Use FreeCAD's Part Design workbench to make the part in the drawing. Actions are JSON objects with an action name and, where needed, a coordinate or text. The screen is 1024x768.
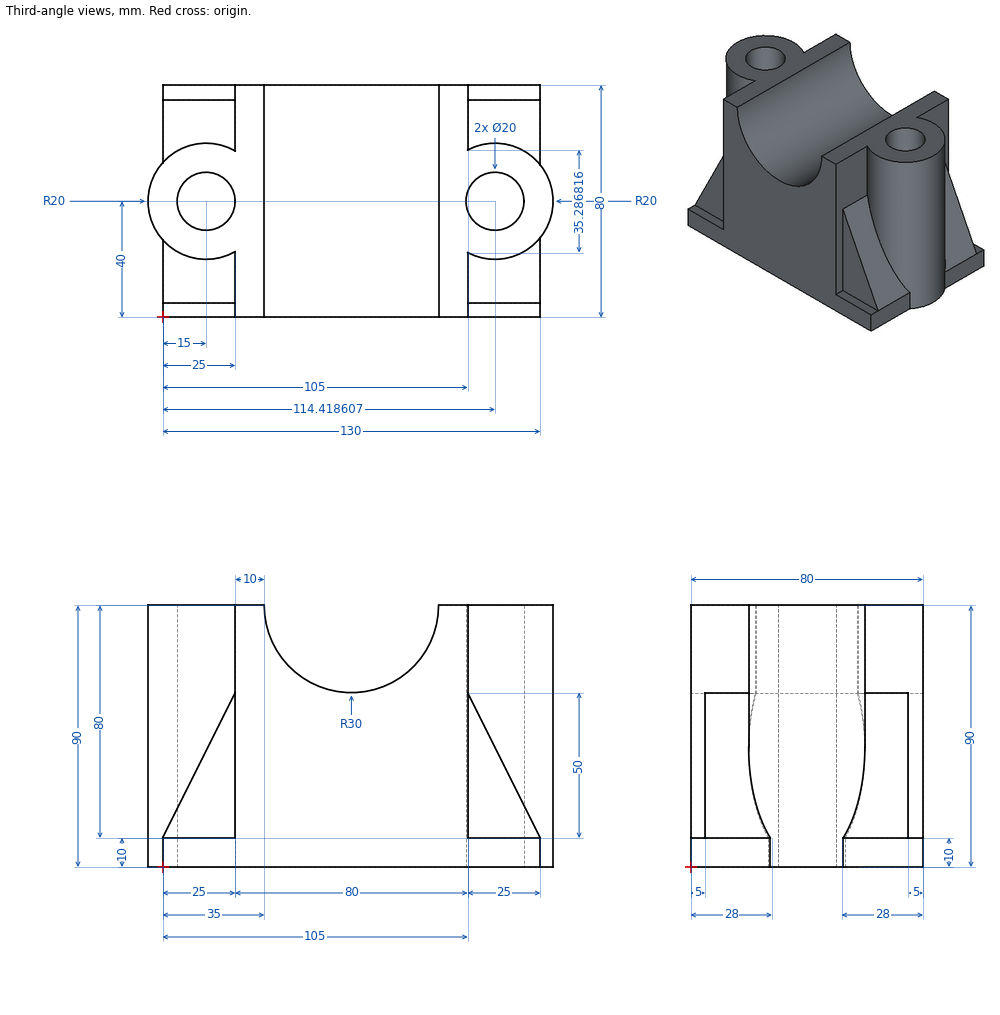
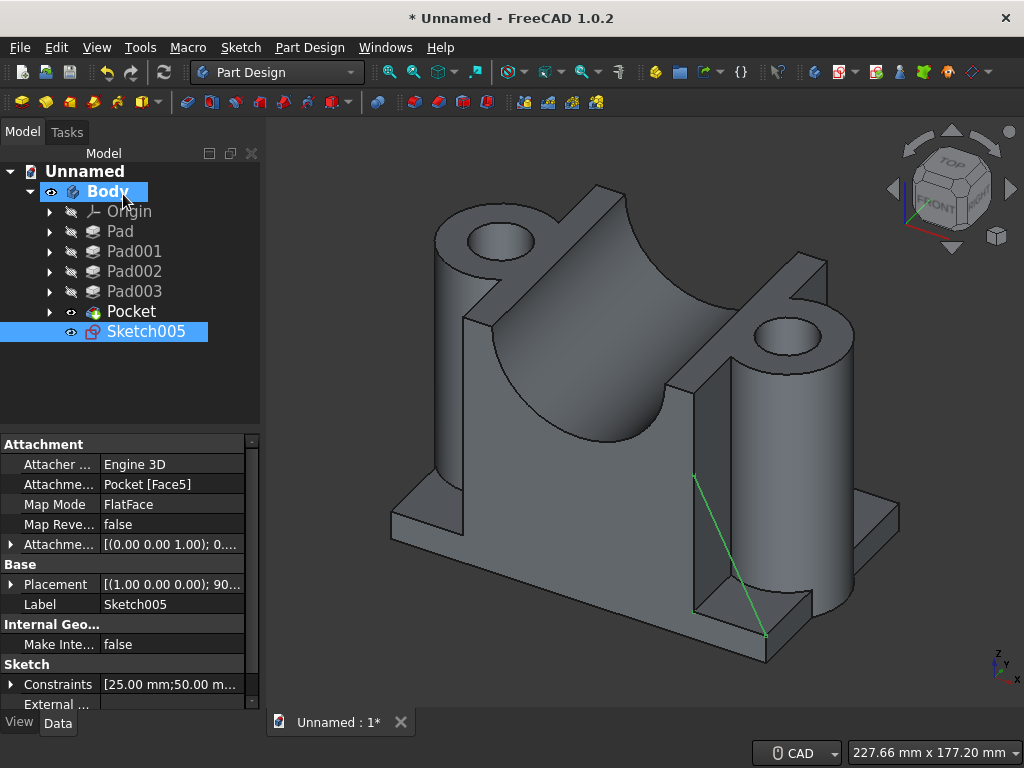
{"action": "left_click", "coordinate": [22, 102]}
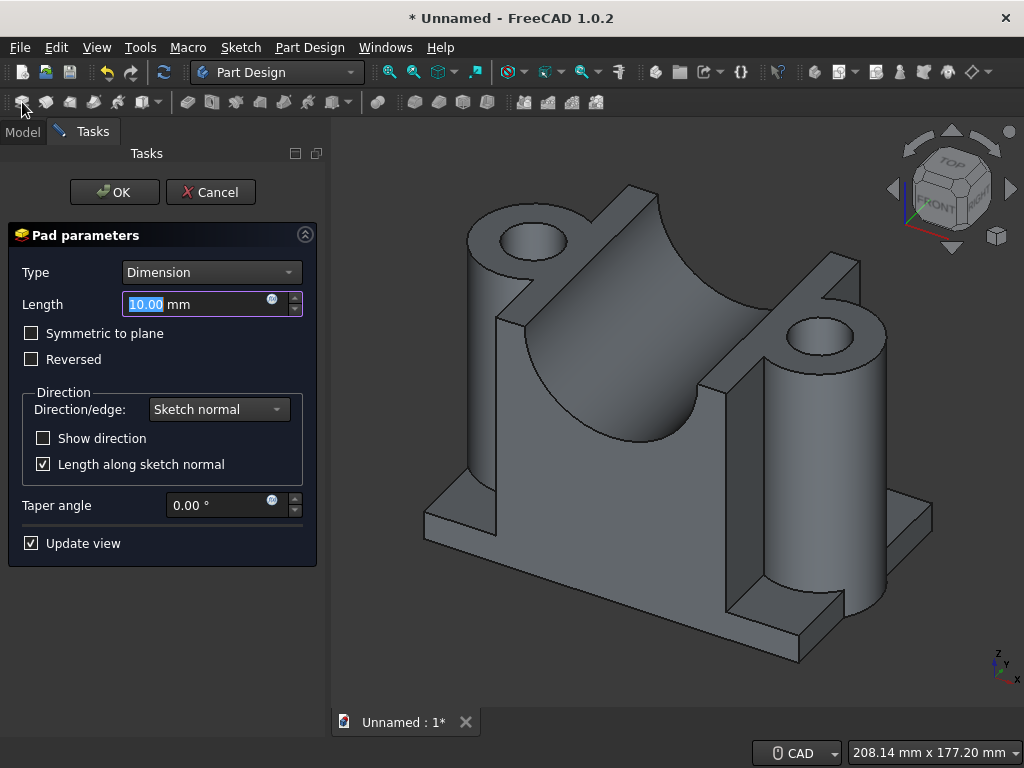
{"action": "type", "text": "28"}
{"action": "key", "text": "Tab"}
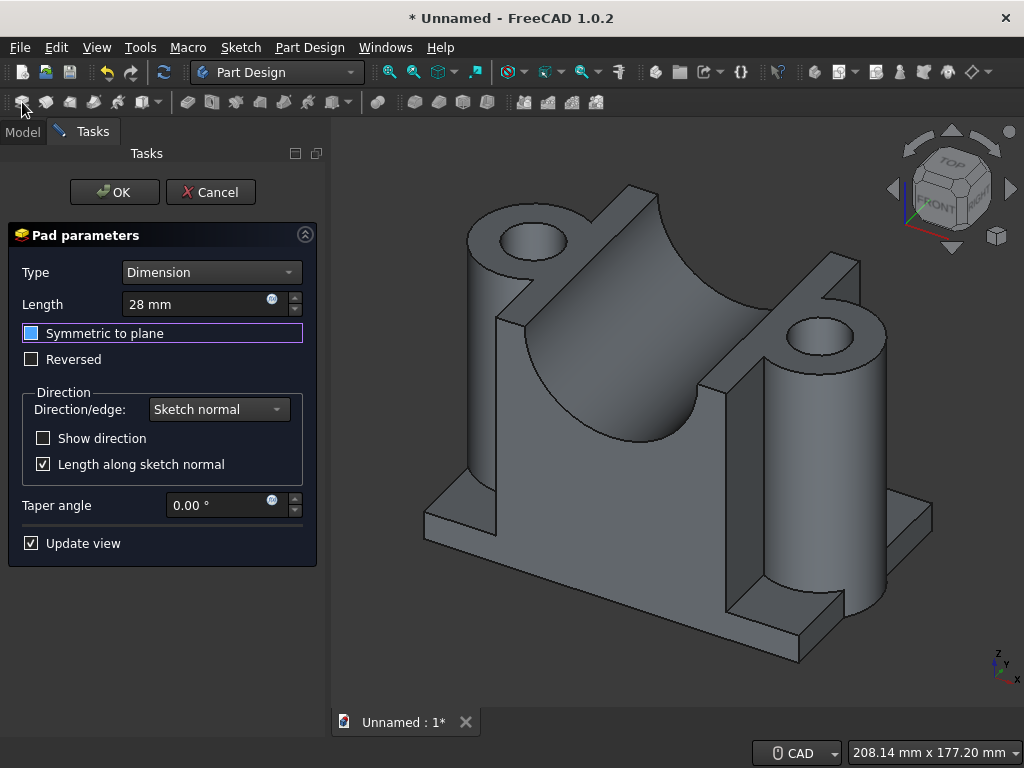
{"action": "left_click", "coordinate": [30, 359]}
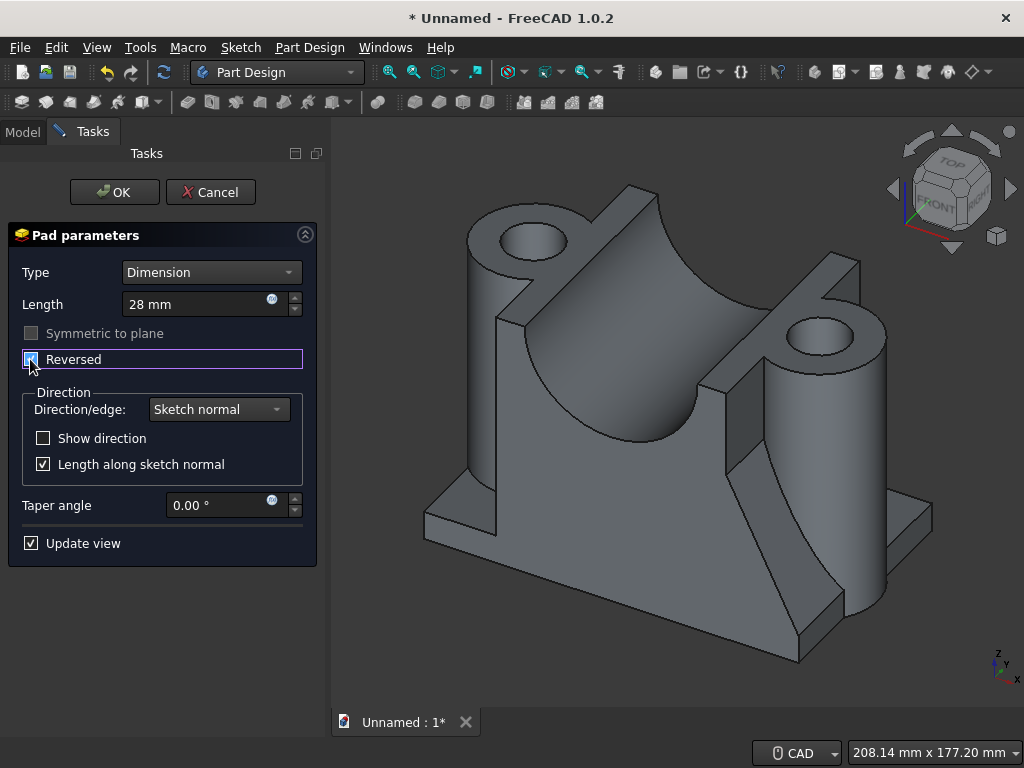
{"action": "left_click", "coordinate": [115, 192]}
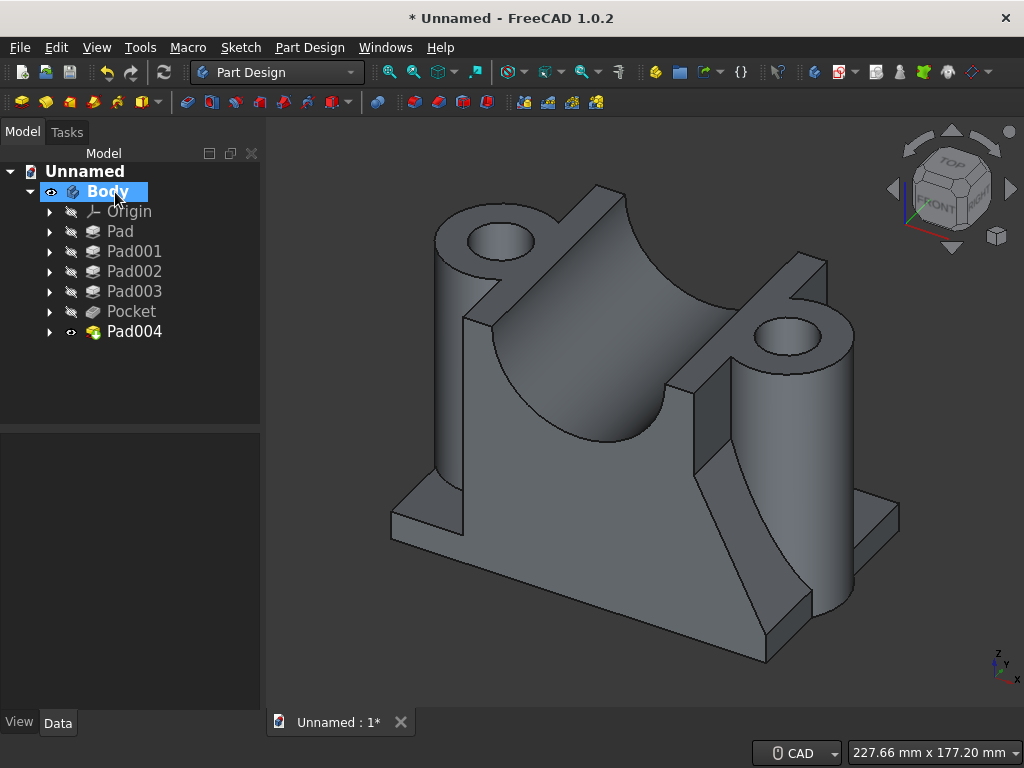
{"action": "left_click", "coordinate": [840, 72]}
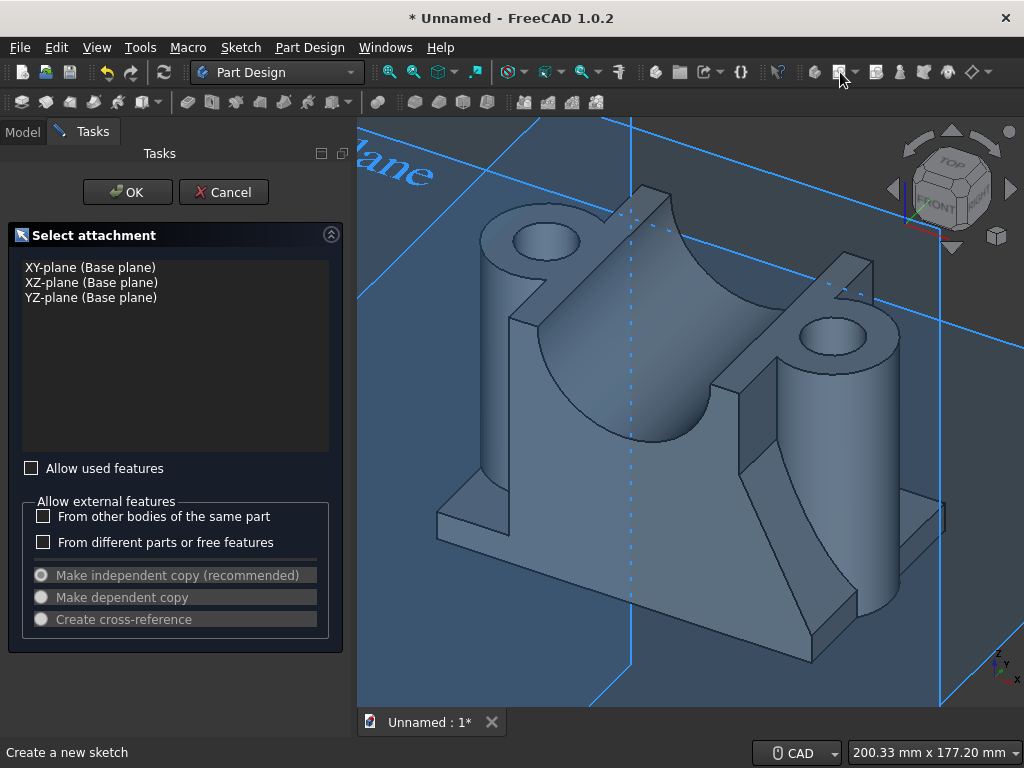
{"action": "left_click", "coordinate": [82, 282]}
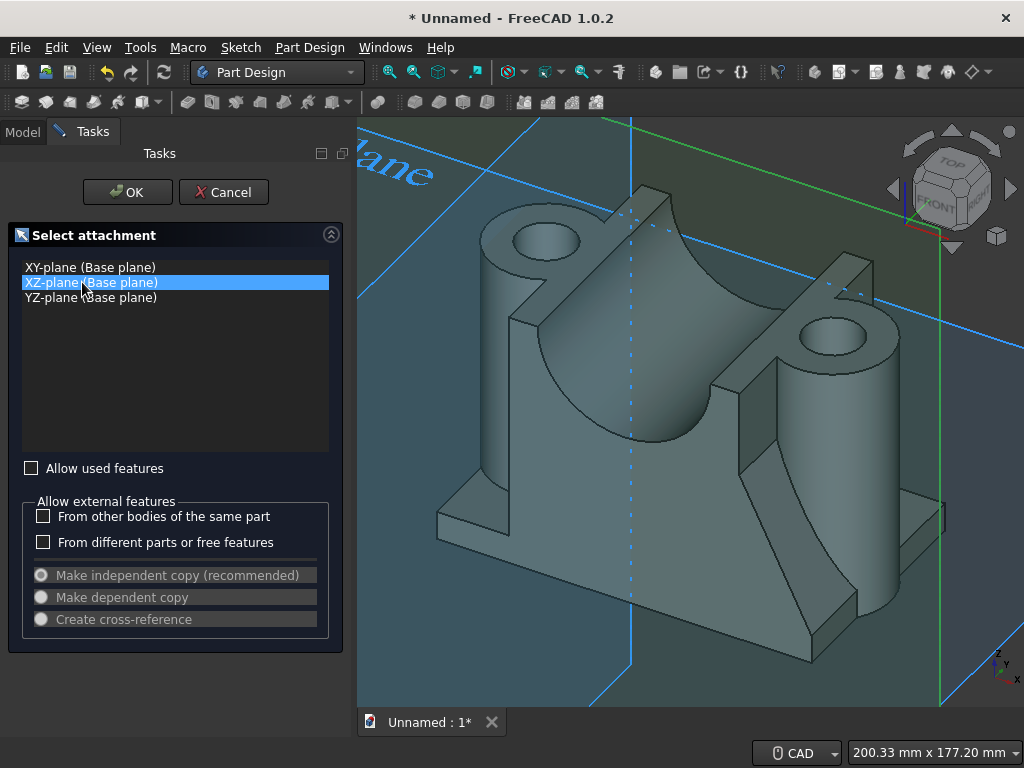
{"action": "left_click", "coordinate": [128, 192]}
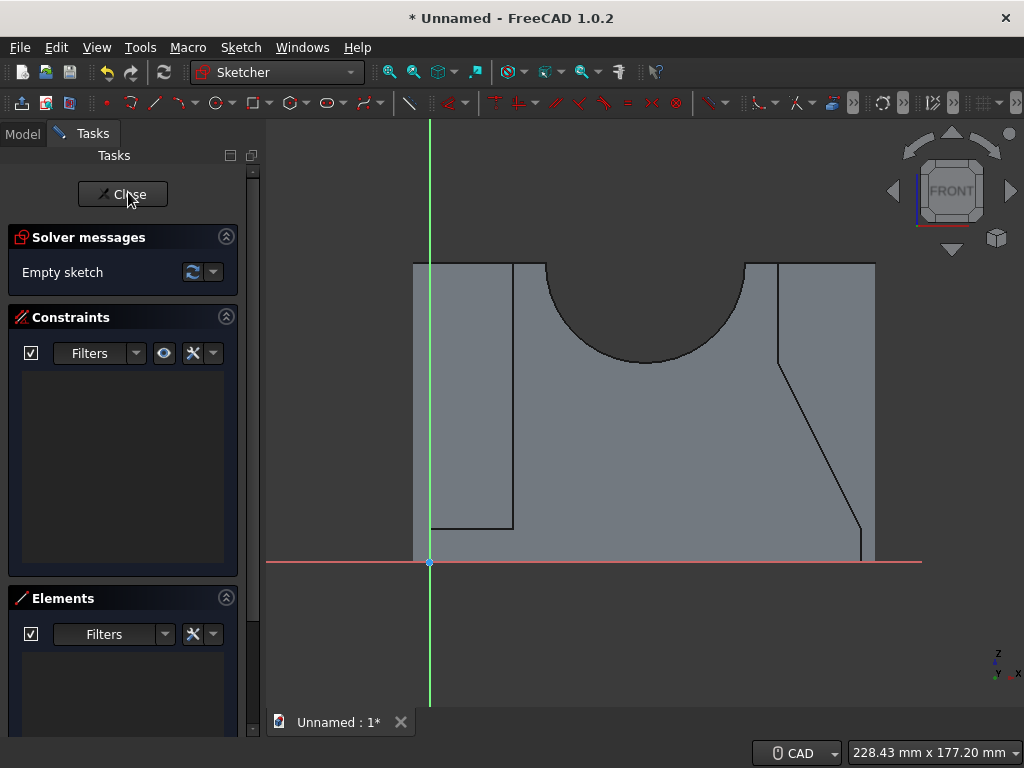
{"action": "scroll", "coordinate": [343, 523], "scroll_direction": "up", "scroll_amount": 3}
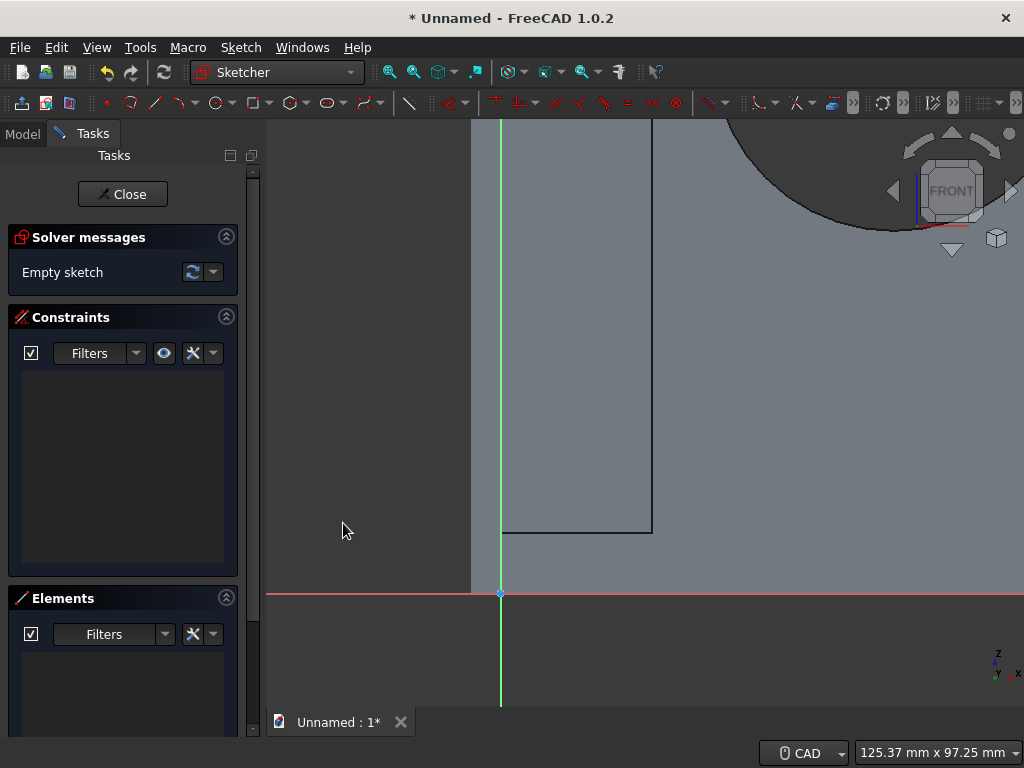
{"action": "left_click", "coordinate": [132, 104]}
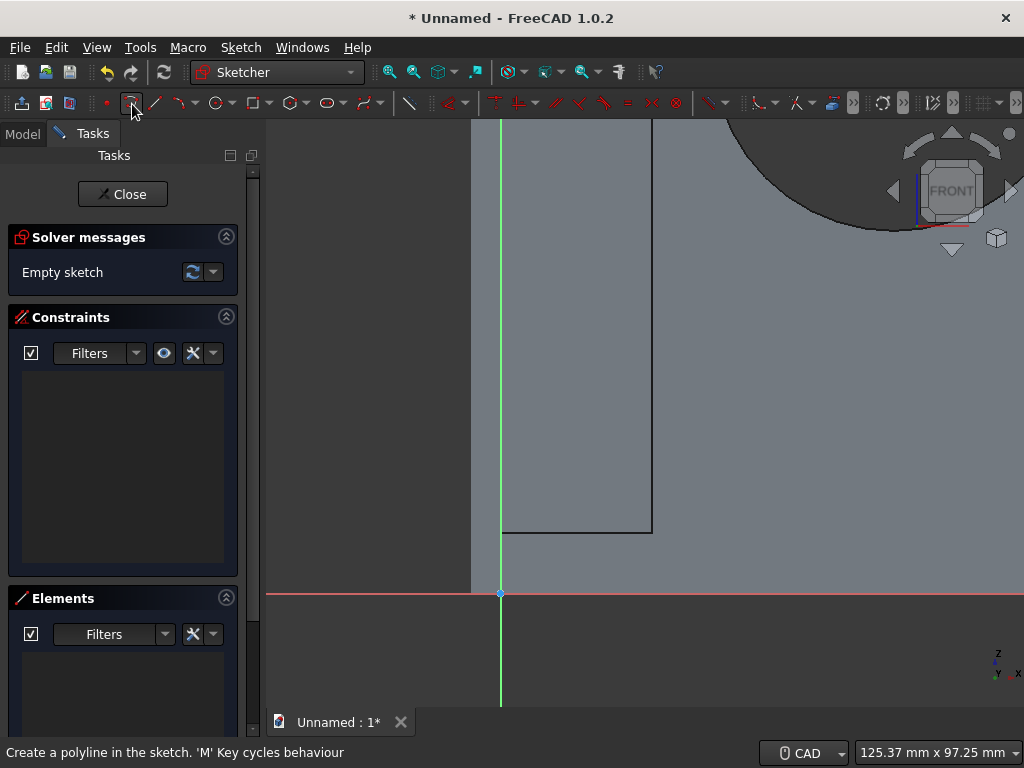
{"action": "left_click", "coordinate": [501, 533]}
{"action": "left_click", "coordinate": [652, 533]}
{"action": "left_click", "coordinate": [652, 231]}
{"action": "left_click", "coordinate": [501, 534]}
{"action": "key", "text": "Escape"}
{"action": "key", "text": "Escape"}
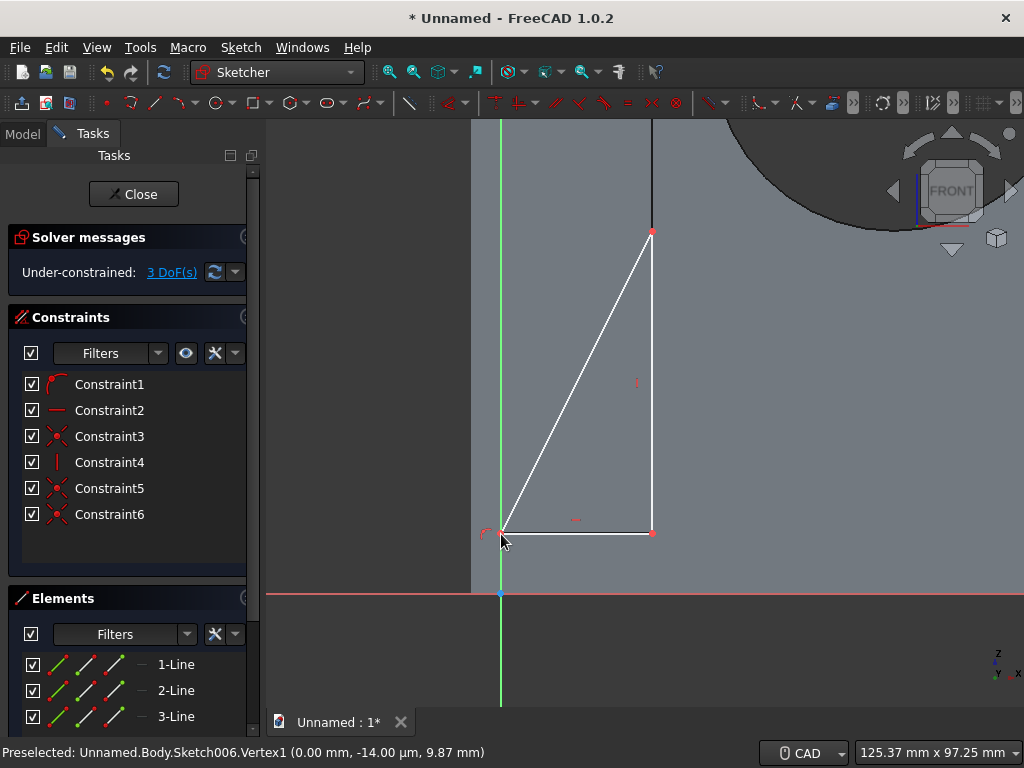
{"action": "left_click", "coordinate": [448, 104]}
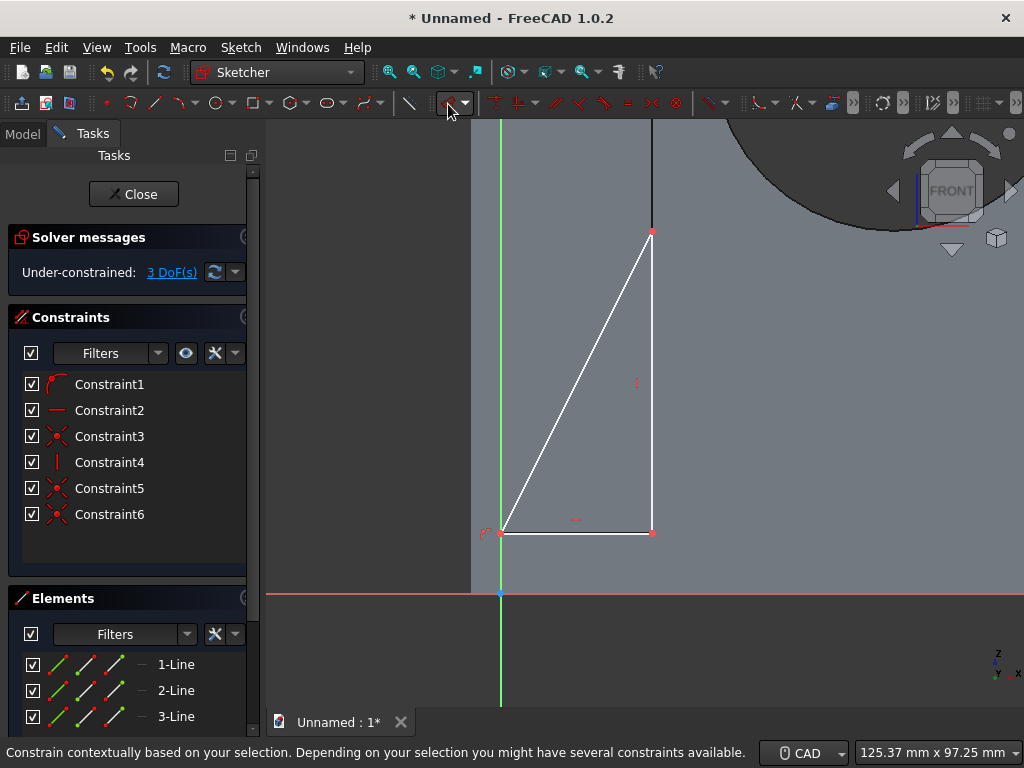
{"action": "left_click", "coordinate": [546, 534]}
{"action": "left_click", "coordinate": [576, 568]}